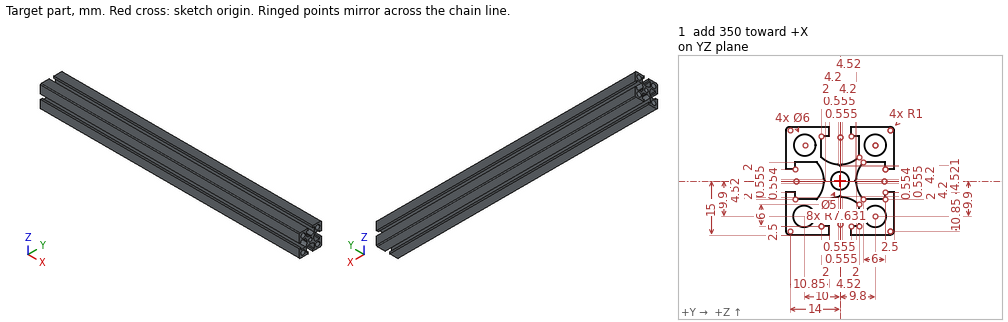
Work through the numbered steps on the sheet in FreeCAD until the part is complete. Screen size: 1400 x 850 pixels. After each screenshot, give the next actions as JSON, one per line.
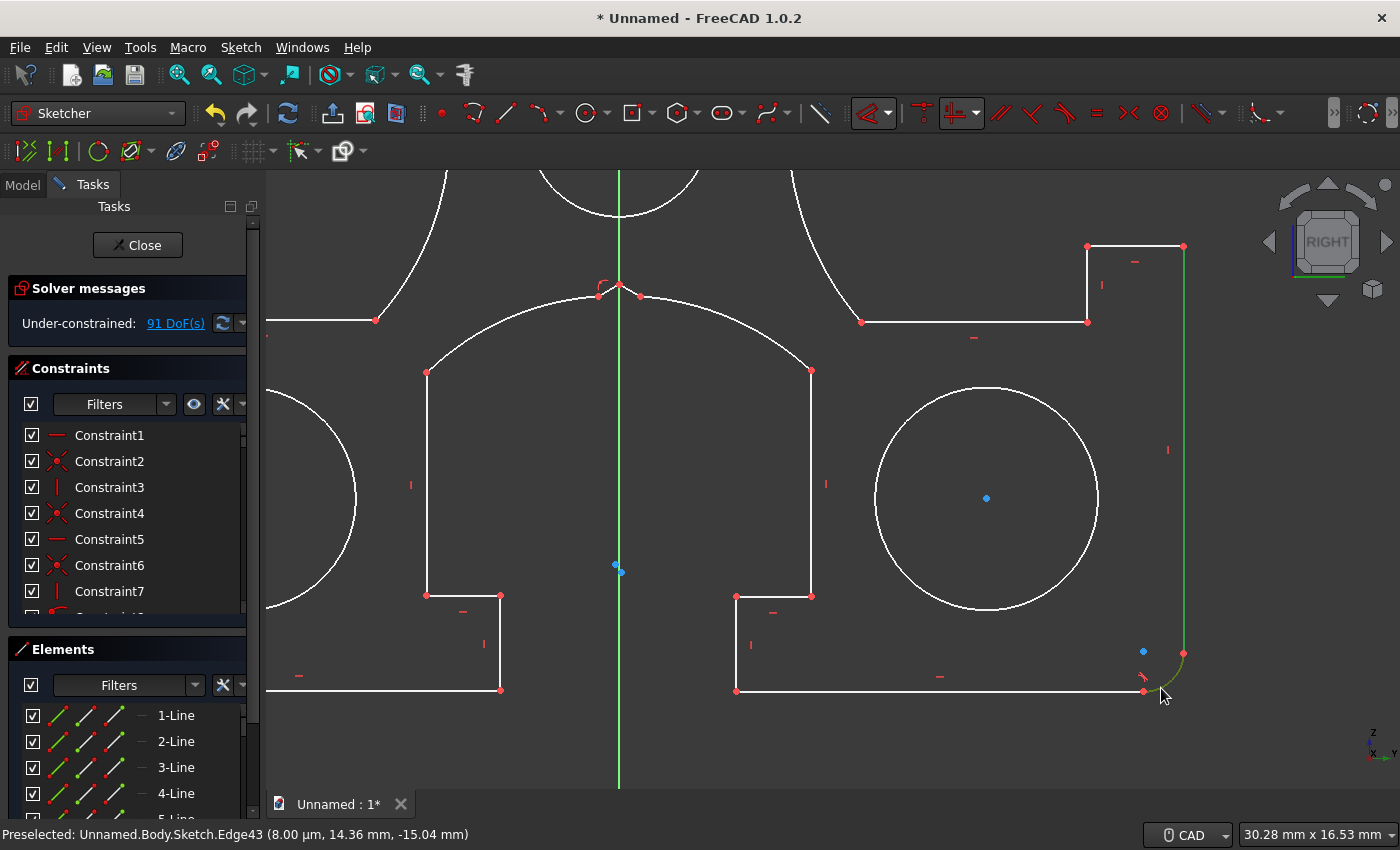
{"action": "left_click", "coordinate": [1066, 114]}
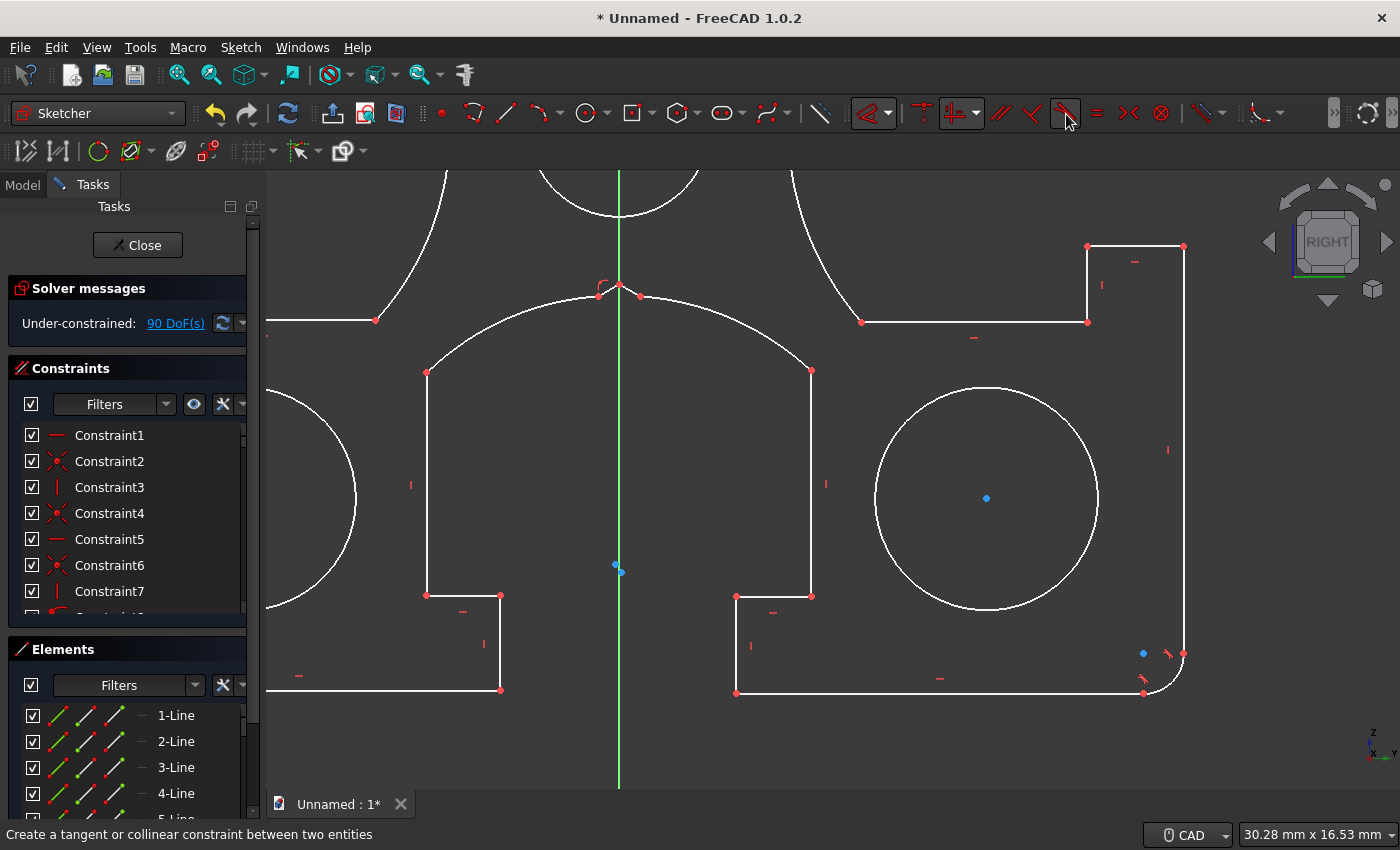
{"action": "scroll", "coordinate": [849, 685], "scroll_direction": "down", "scroll_amount": 5}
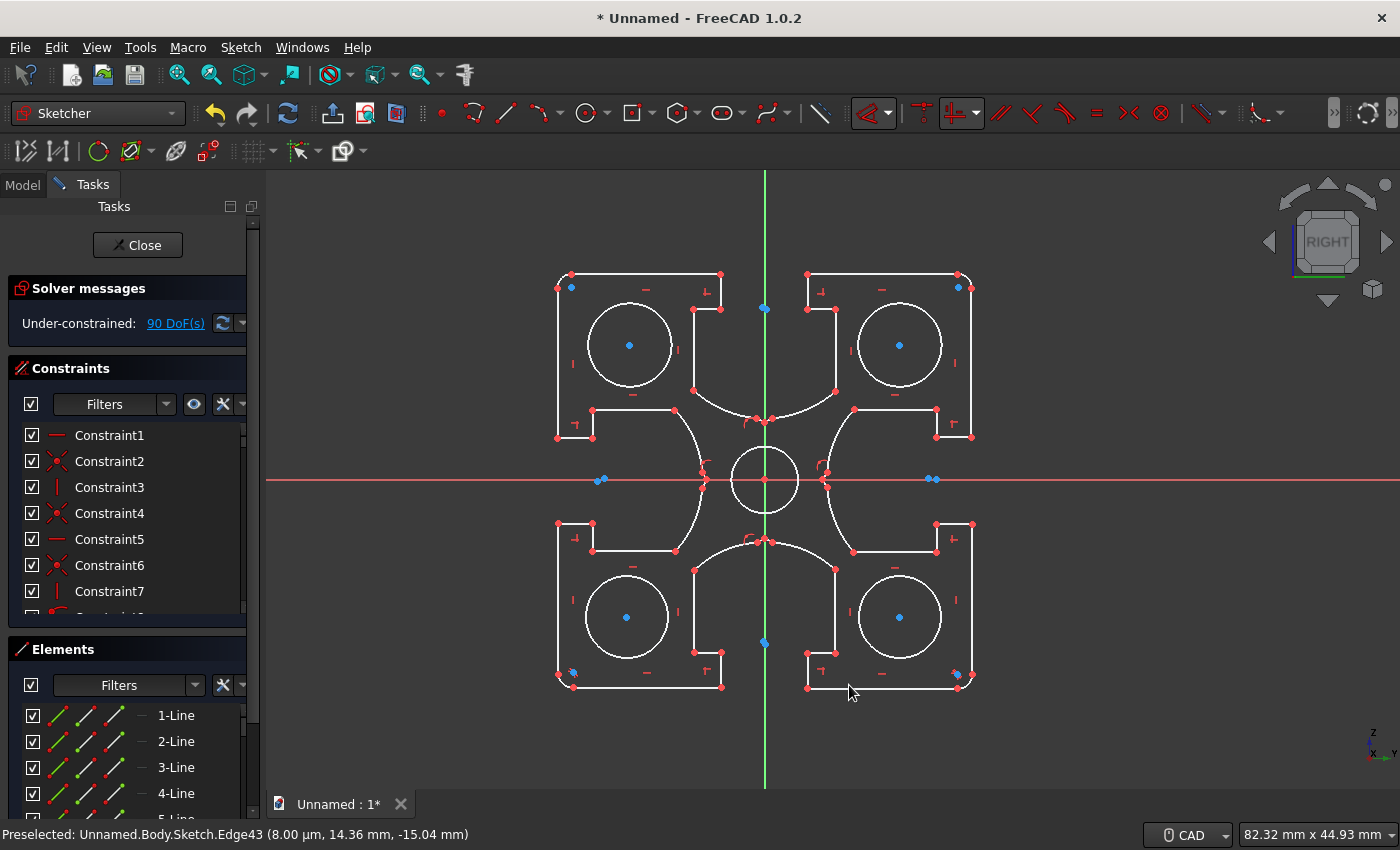
{"action": "left_click", "coordinate": [971, 392]}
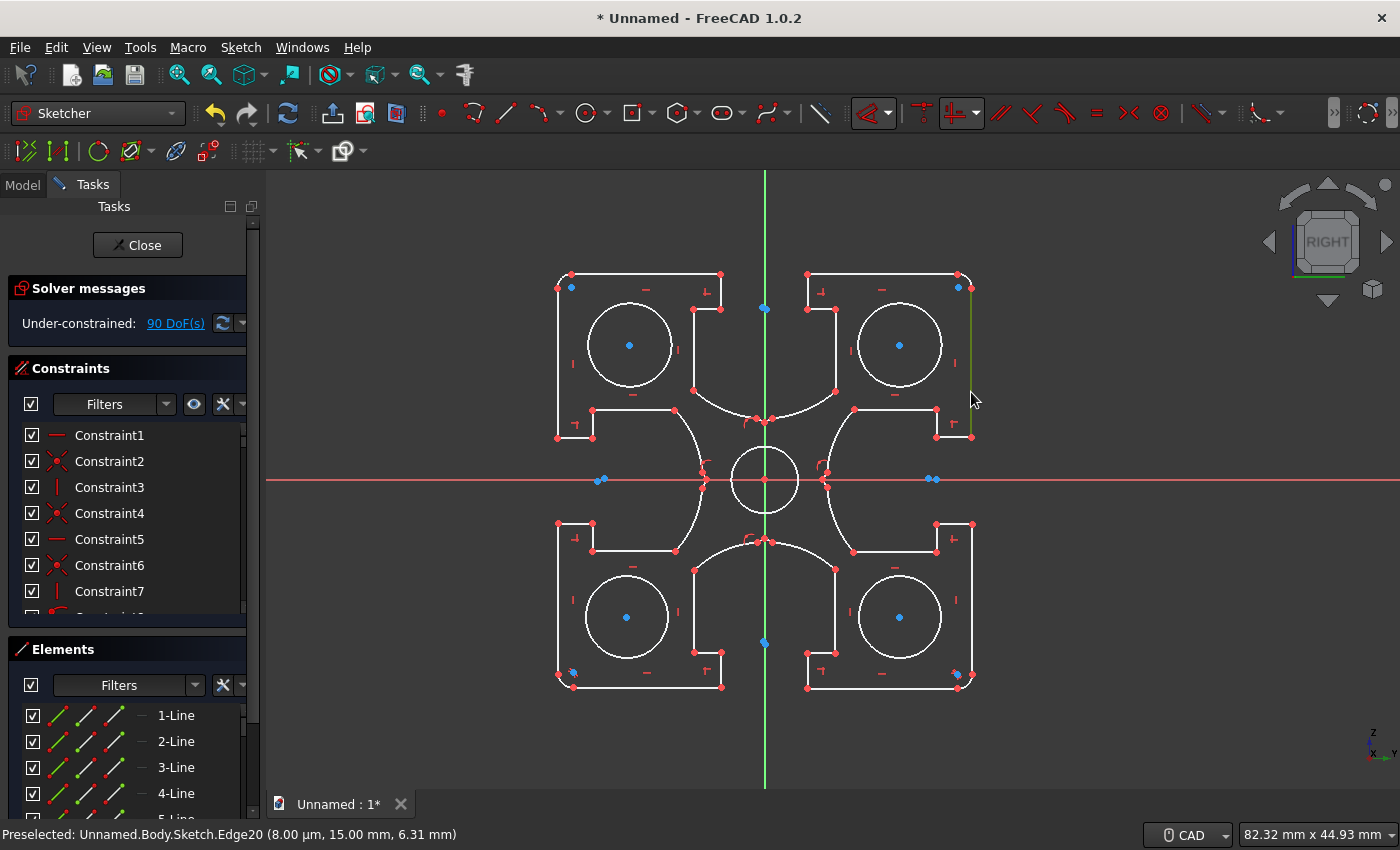
{"action": "scroll", "coordinate": [968, 278], "scroll_direction": "up", "scroll_amount": 2}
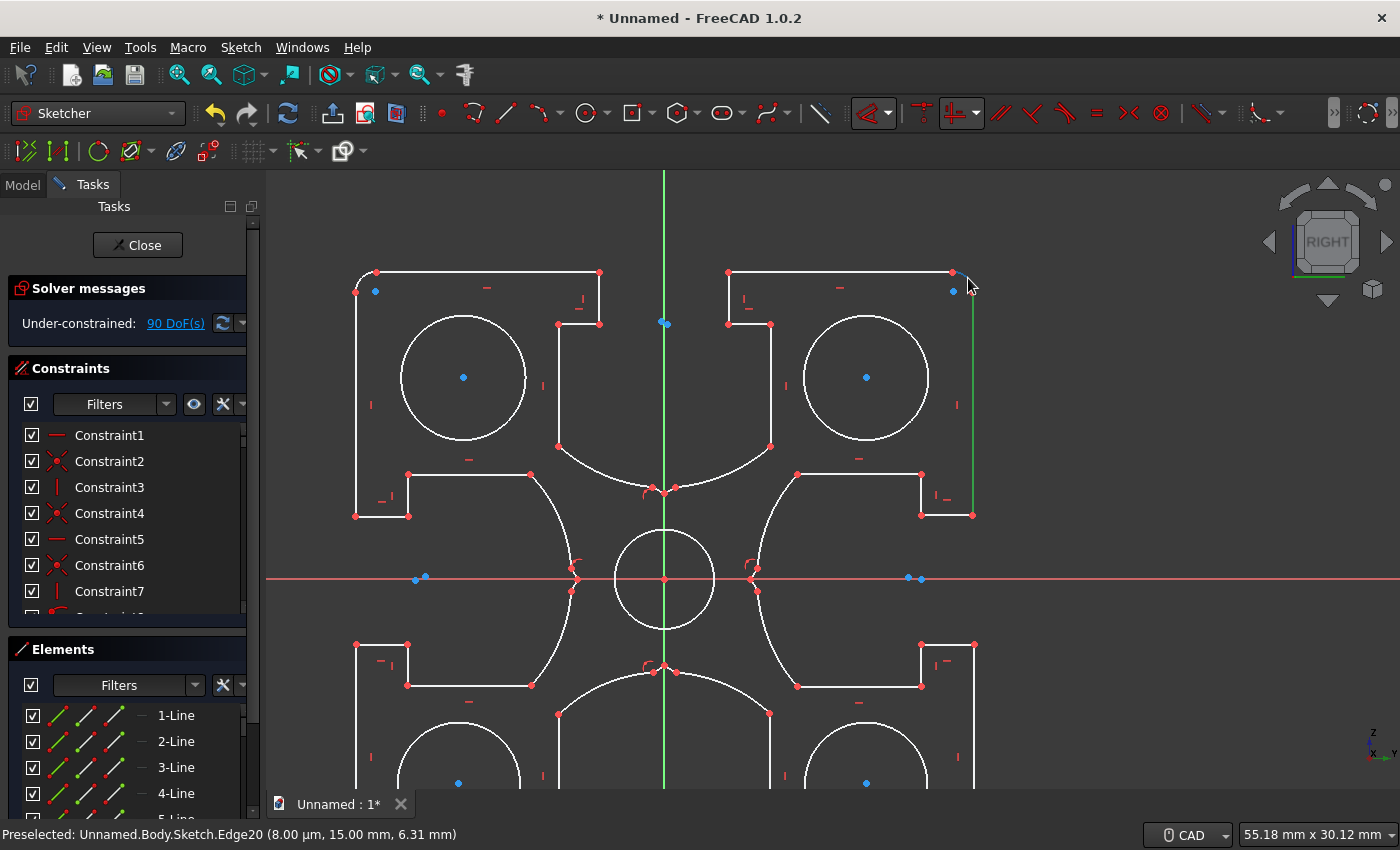
{"action": "left_click", "coordinate": [967, 278]}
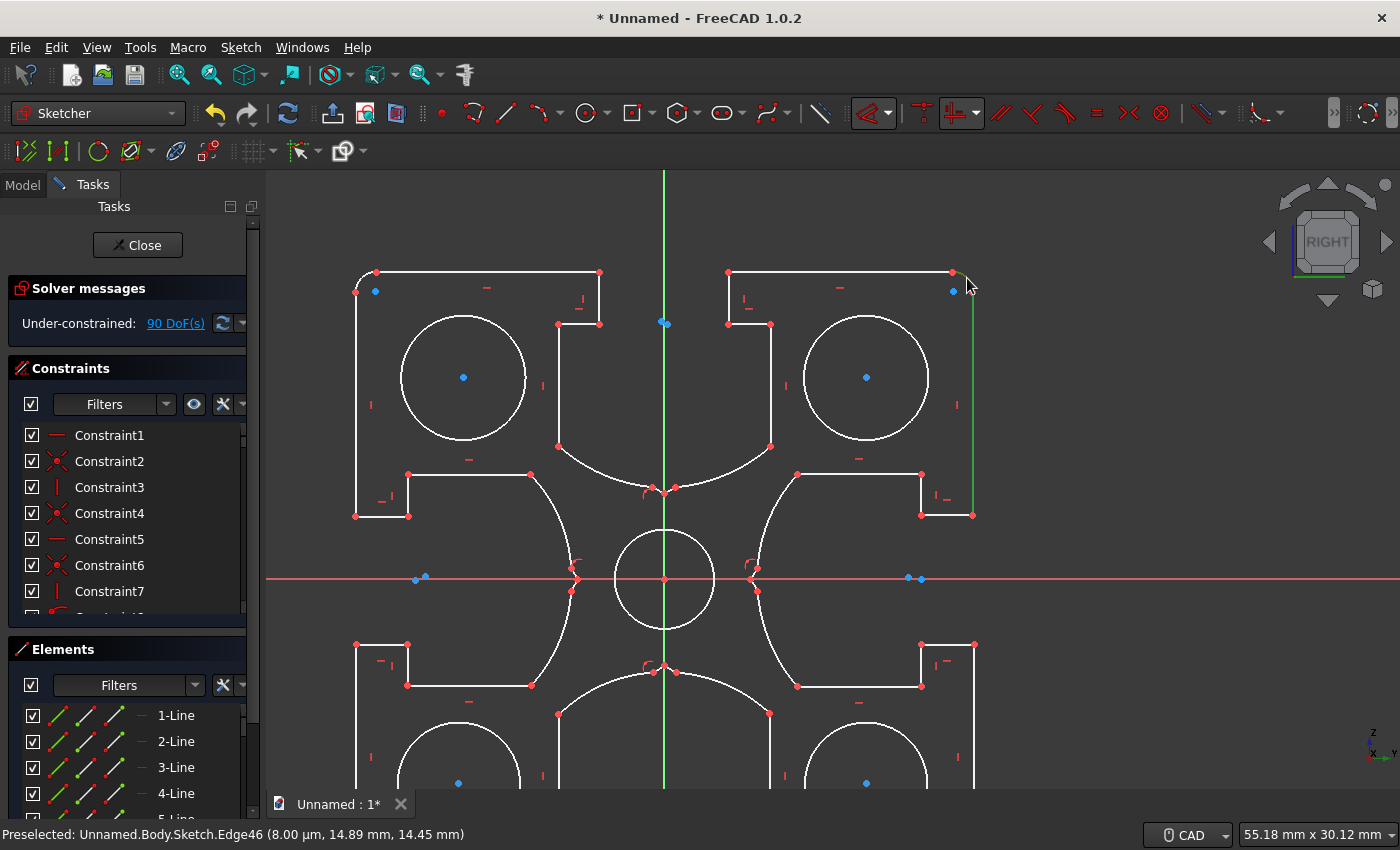
{"action": "left_click", "coordinate": [1066, 114]}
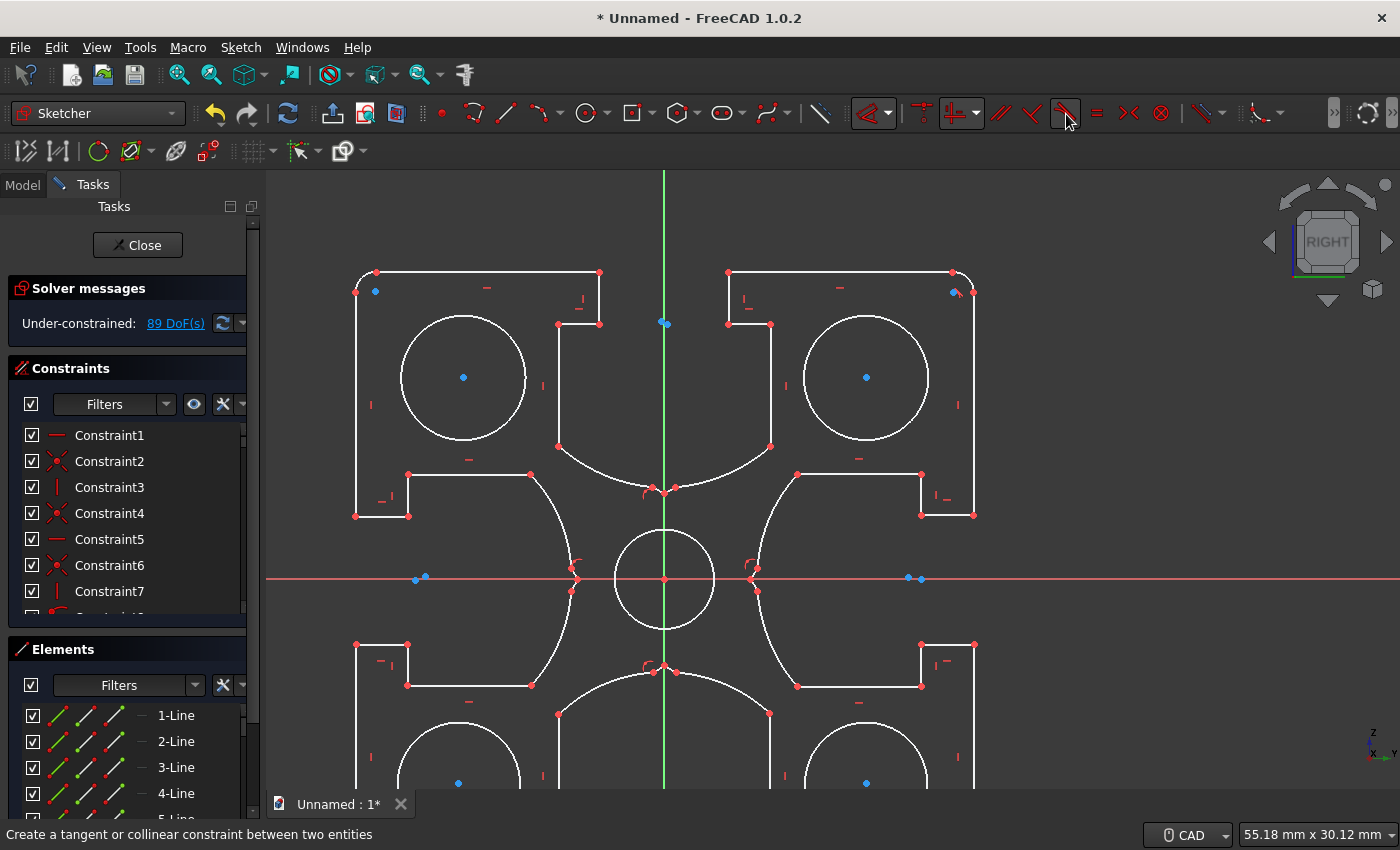
{"action": "left_click", "coordinate": [886, 272]}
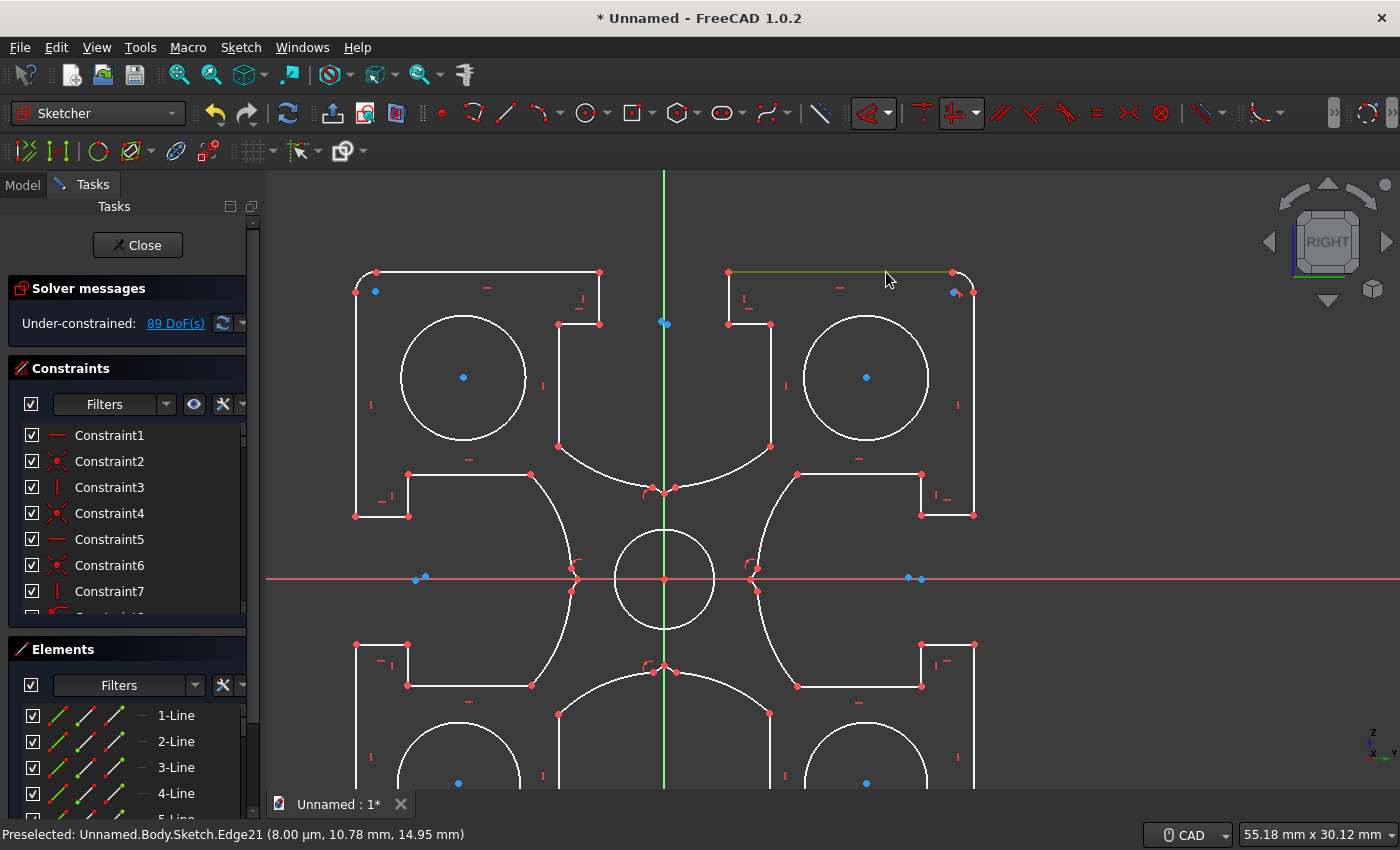
{"action": "scroll", "coordinate": [972, 283], "scroll_direction": "up", "scroll_amount": 2}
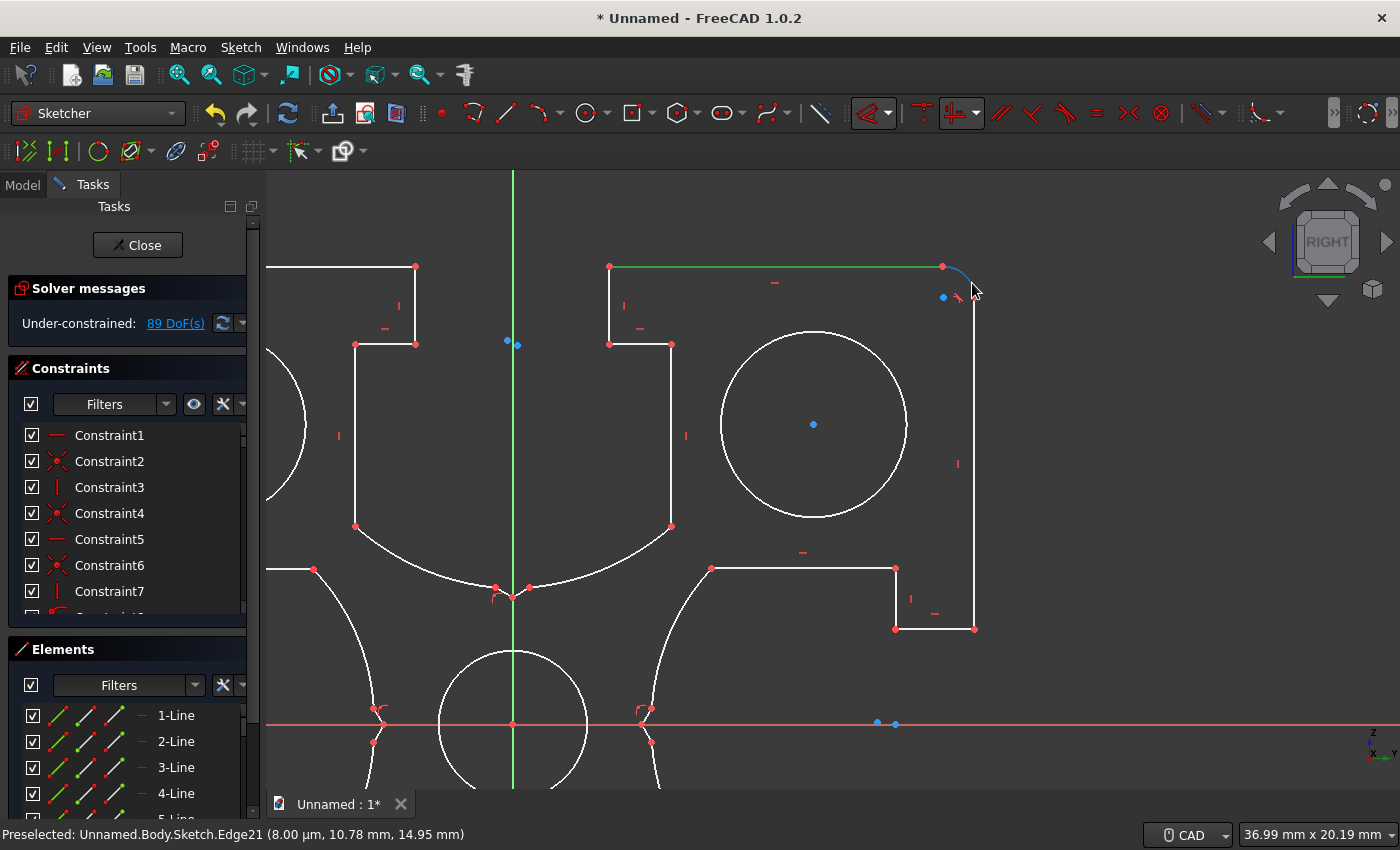
{"action": "left_click", "coordinate": [971, 283]}